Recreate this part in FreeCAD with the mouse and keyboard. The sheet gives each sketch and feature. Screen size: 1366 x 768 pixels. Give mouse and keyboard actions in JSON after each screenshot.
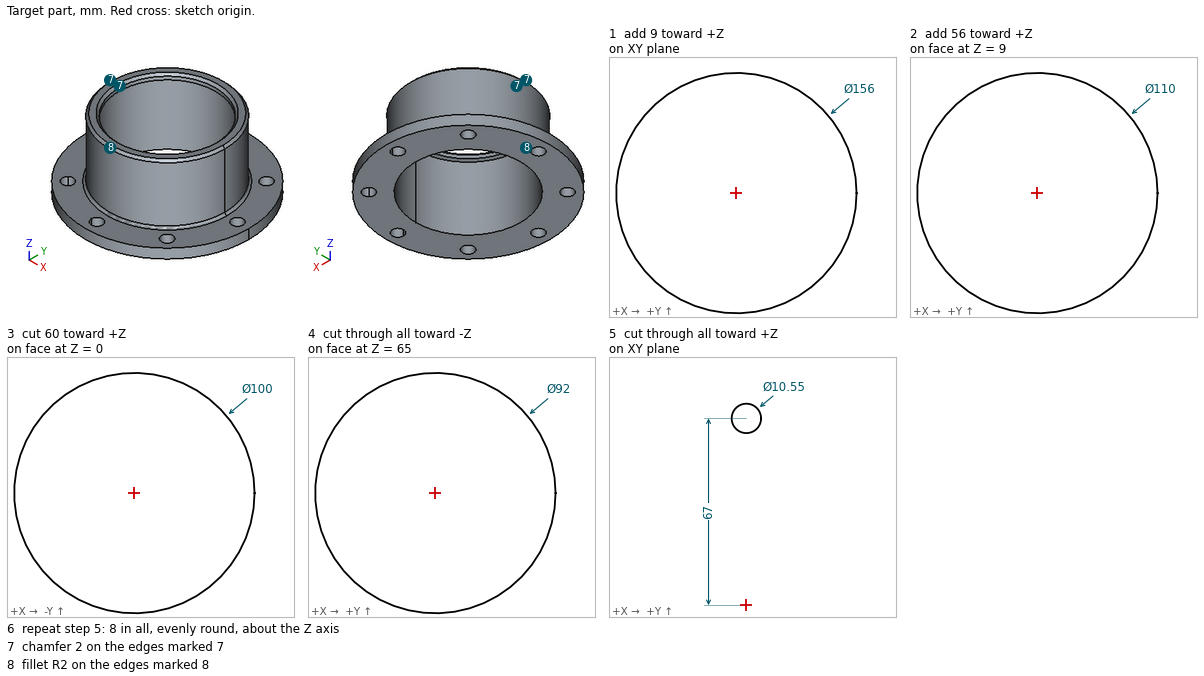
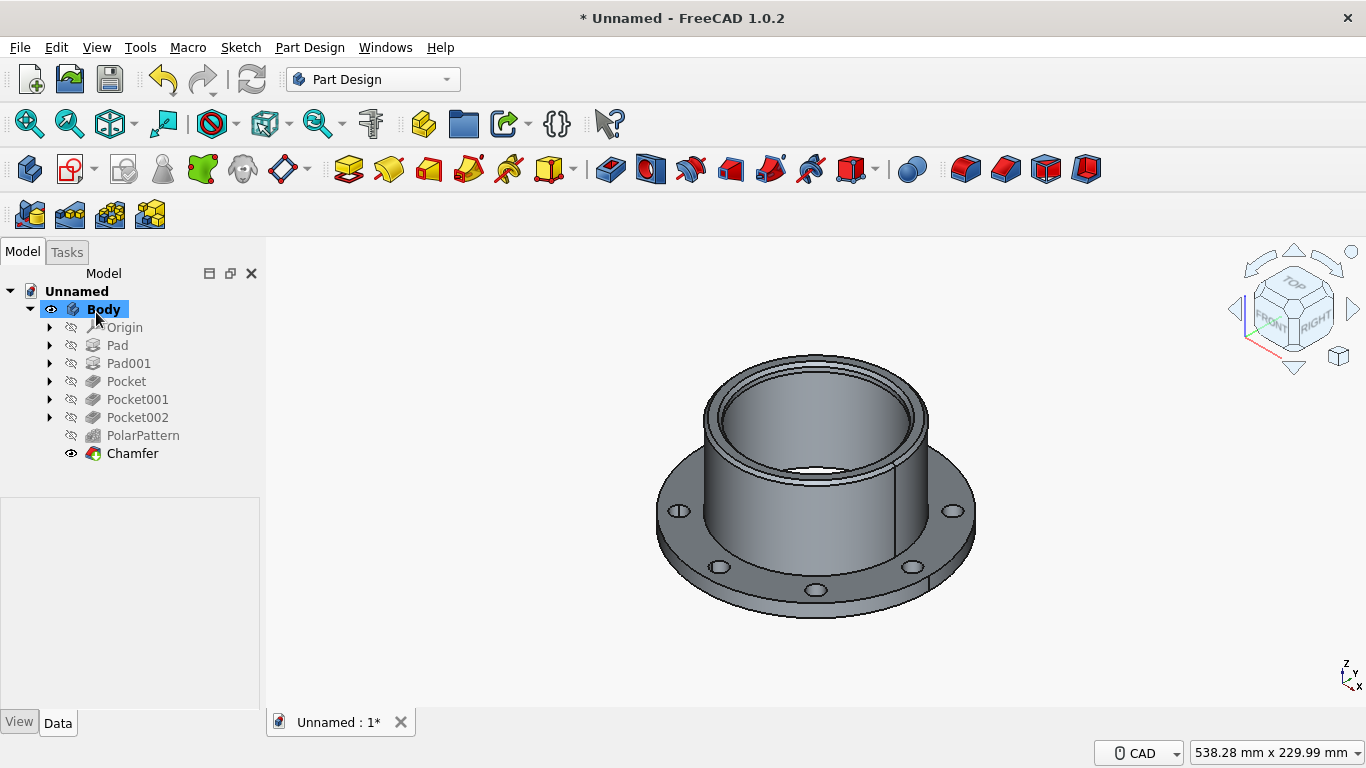
{"action": "key", "text": "1"}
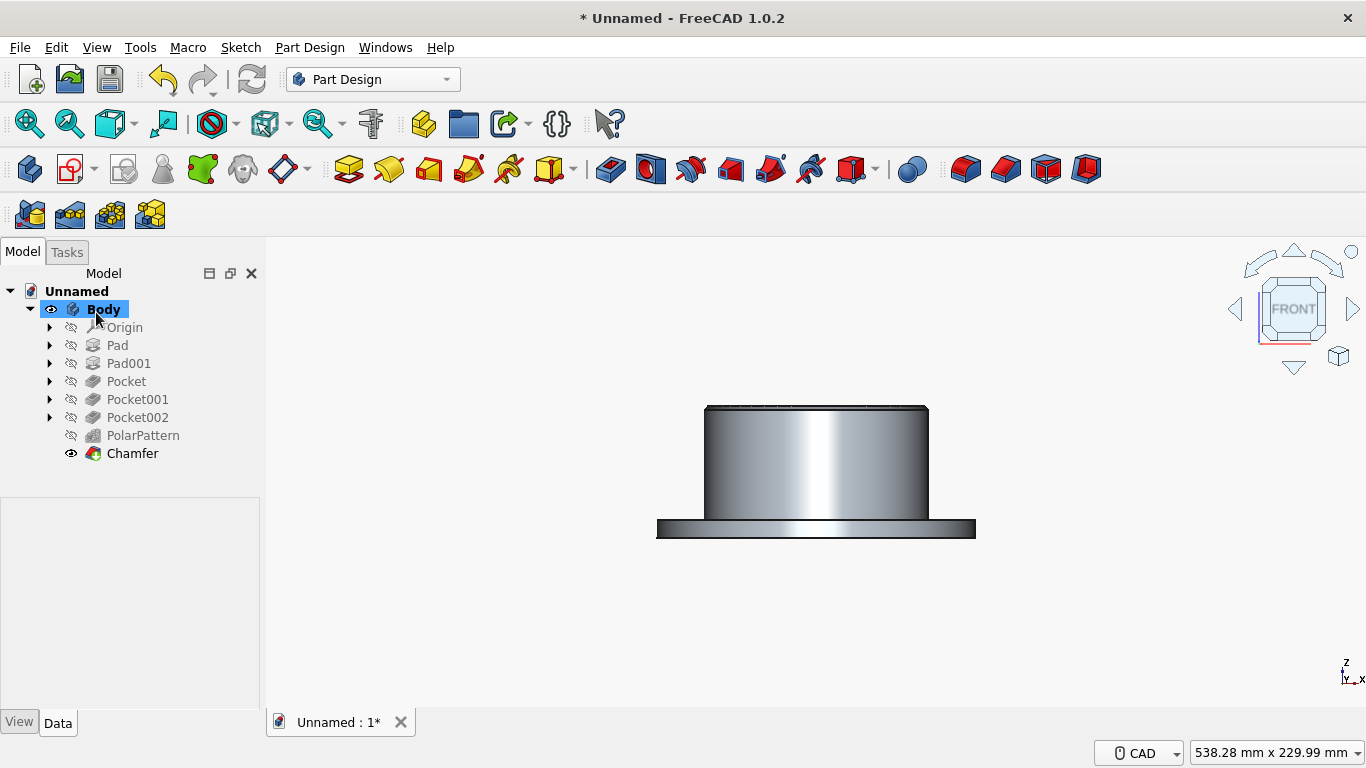
{"action": "left_click", "coordinate": [30, 124]}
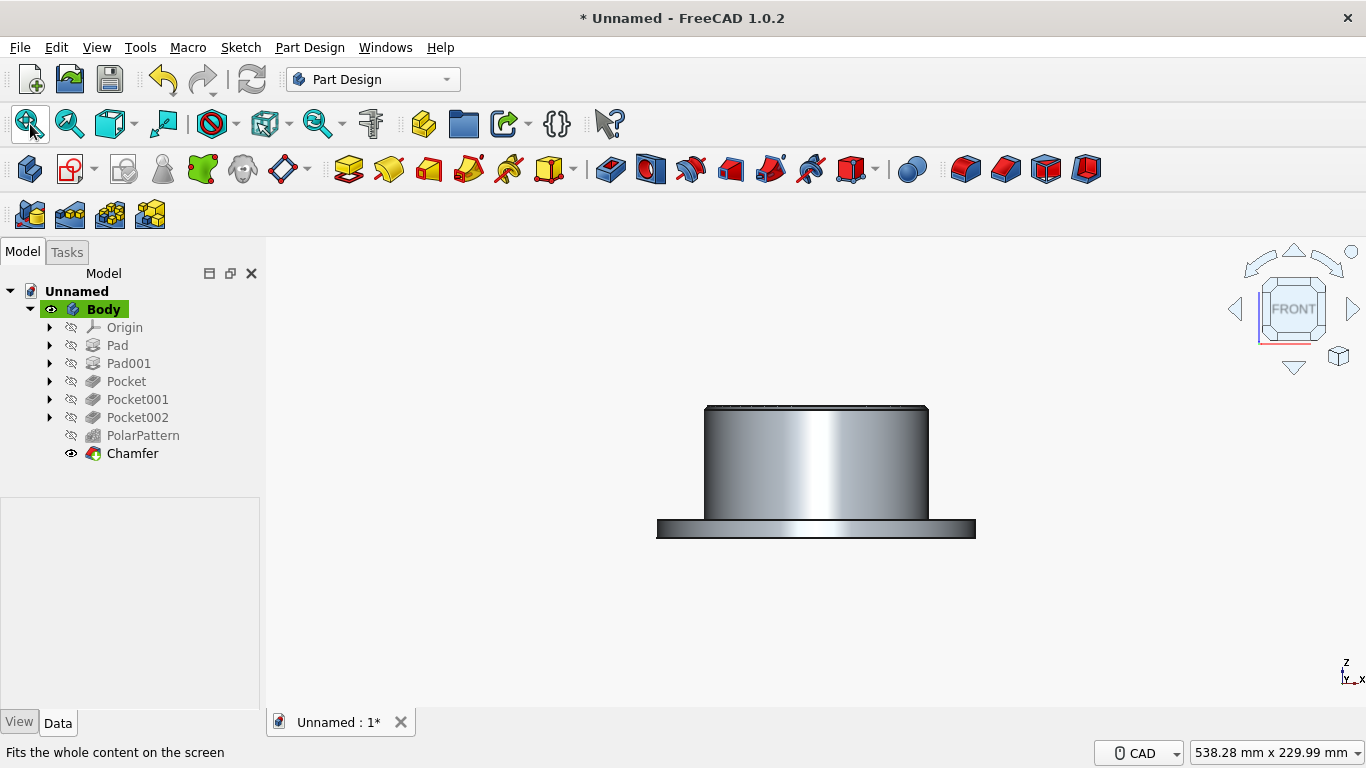
{"action": "key", "text": "3"}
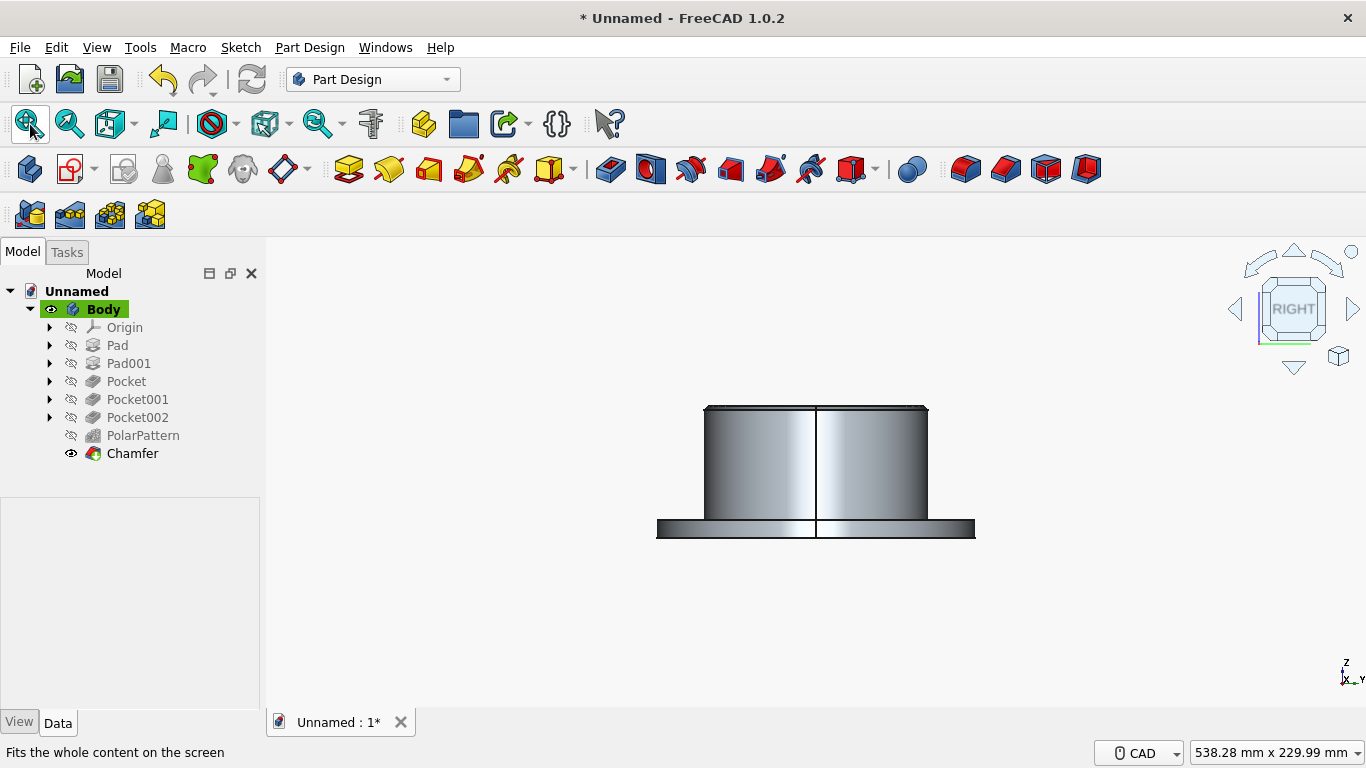
{"action": "left_click", "coordinate": [30, 124]}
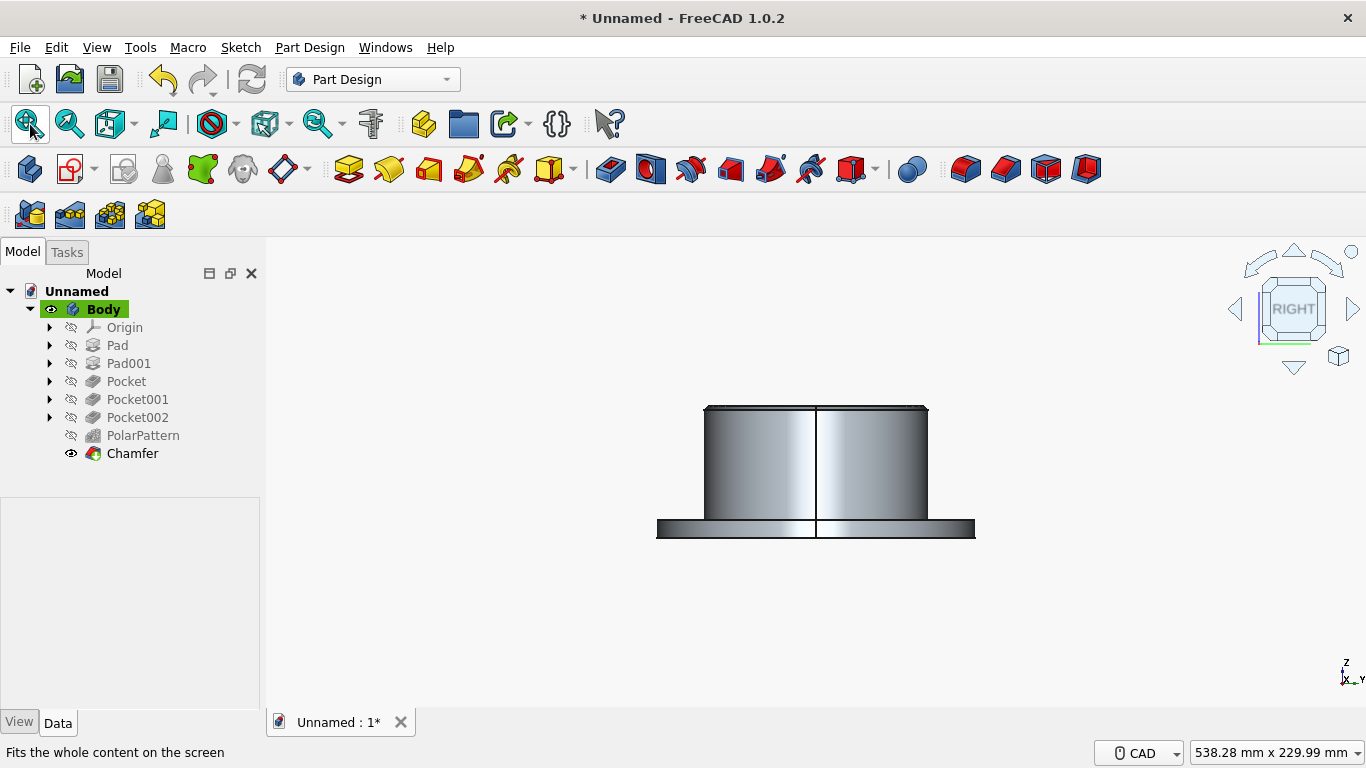
{"action": "key", "text": "5"}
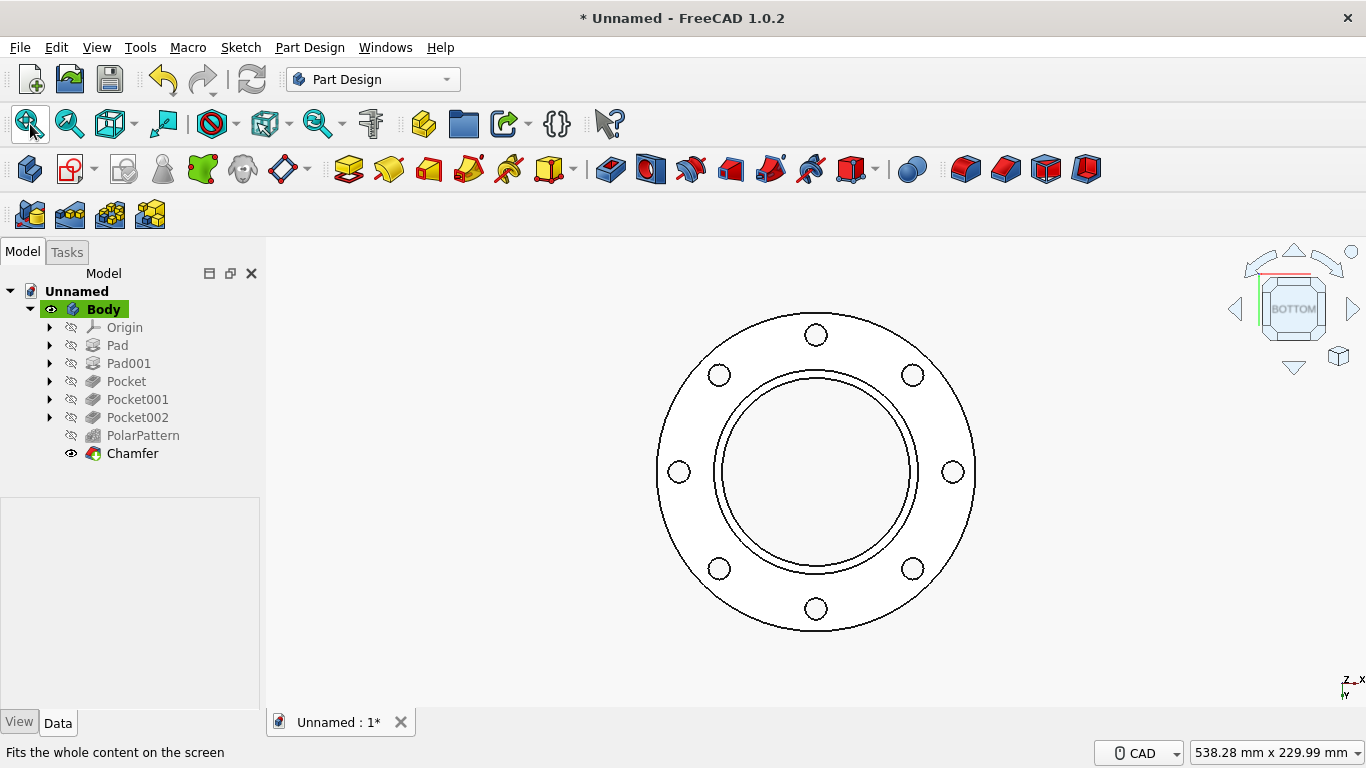
{"action": "key", "text": "4"}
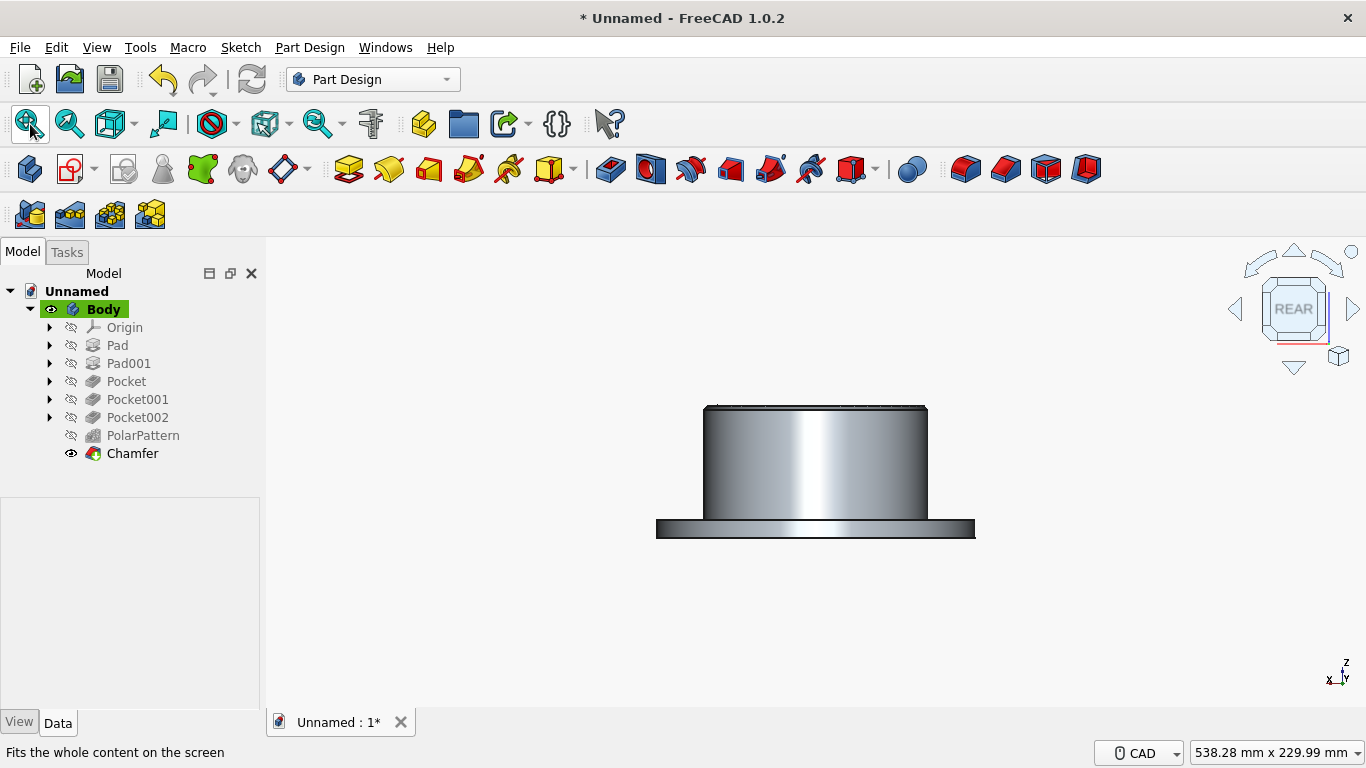
{"action": "key", "text": "v f"}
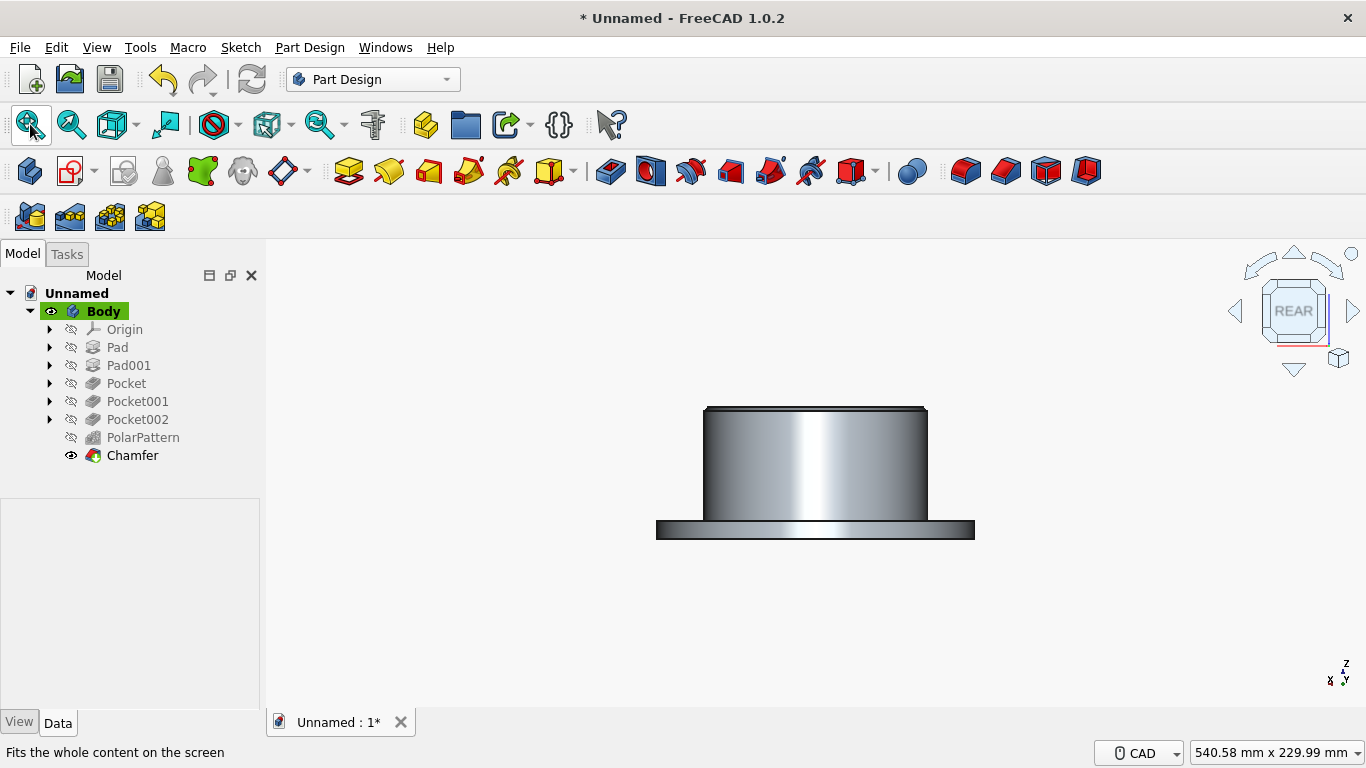
{"action": "key", "text": "6"}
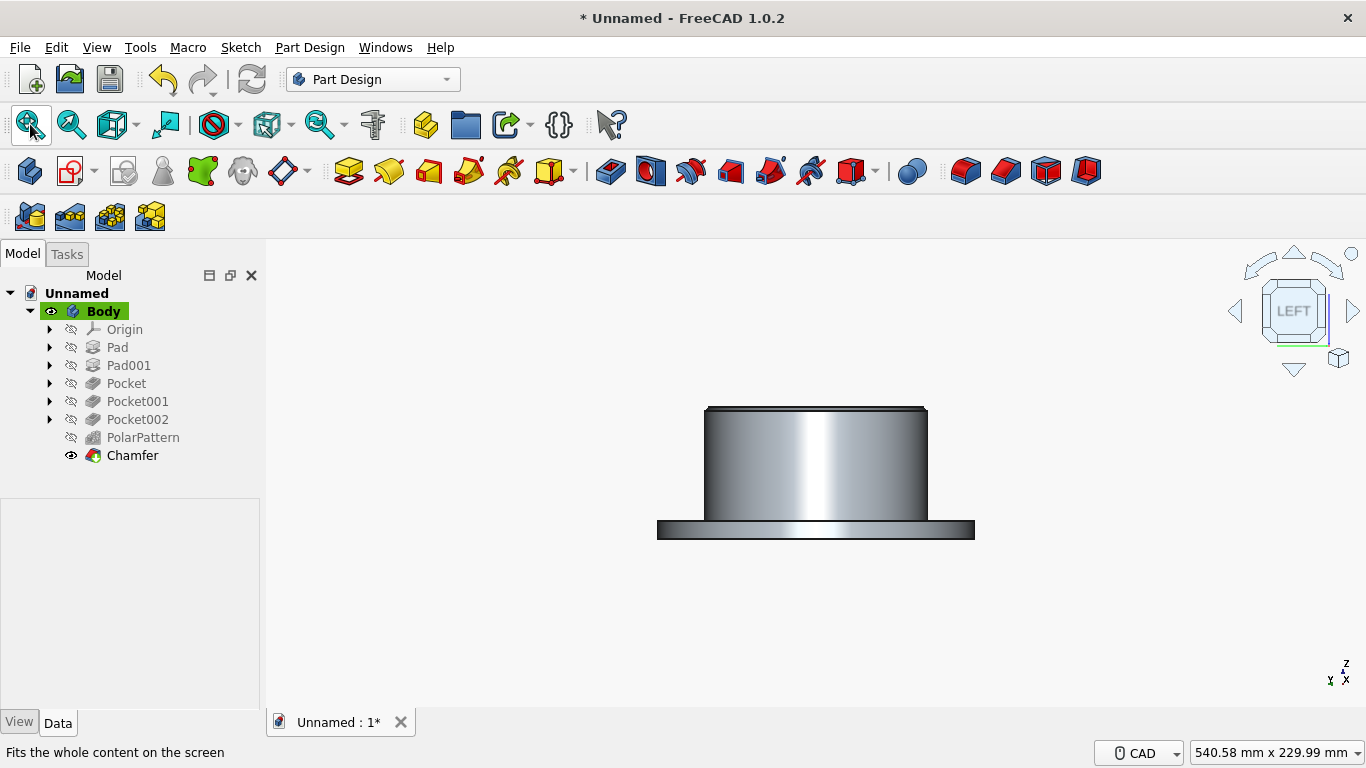
{"action": "key", "text": "v f"}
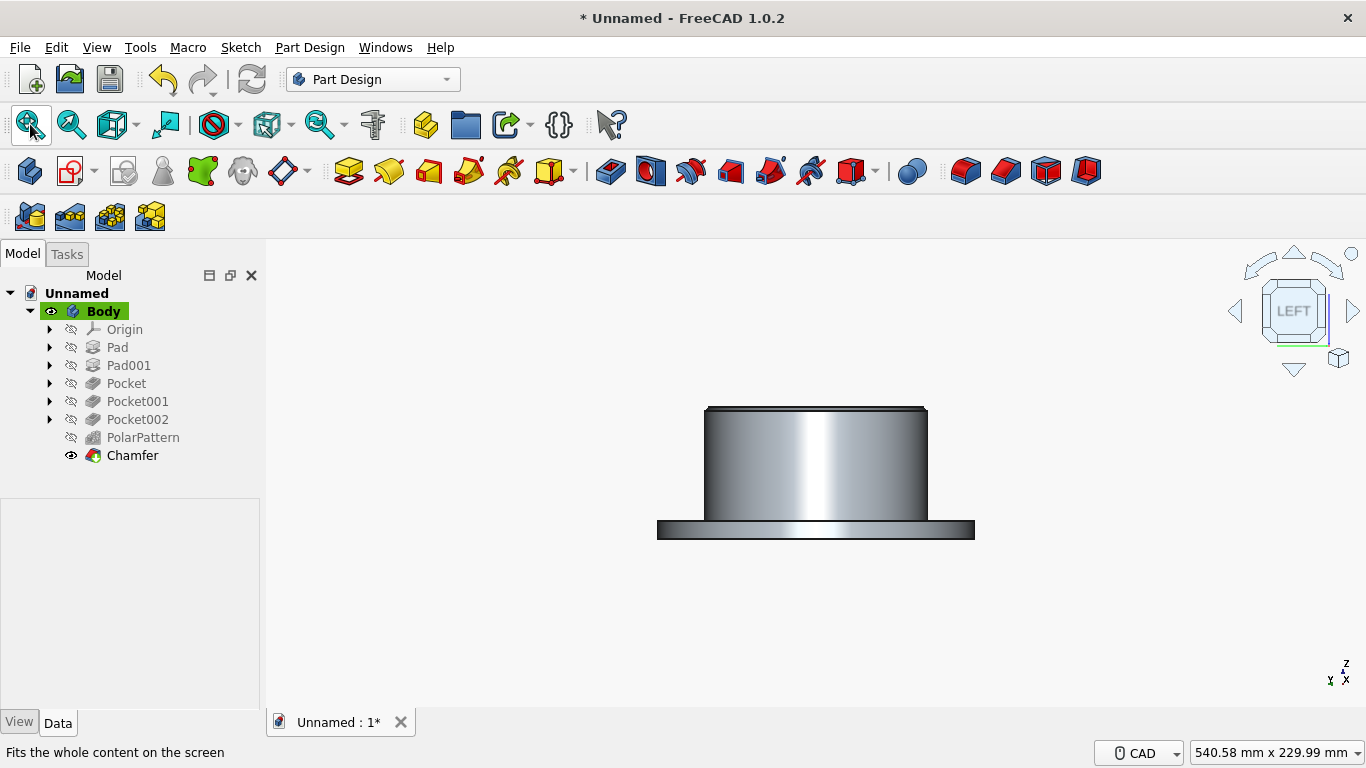
{"action": "key", "text": "v 3"}